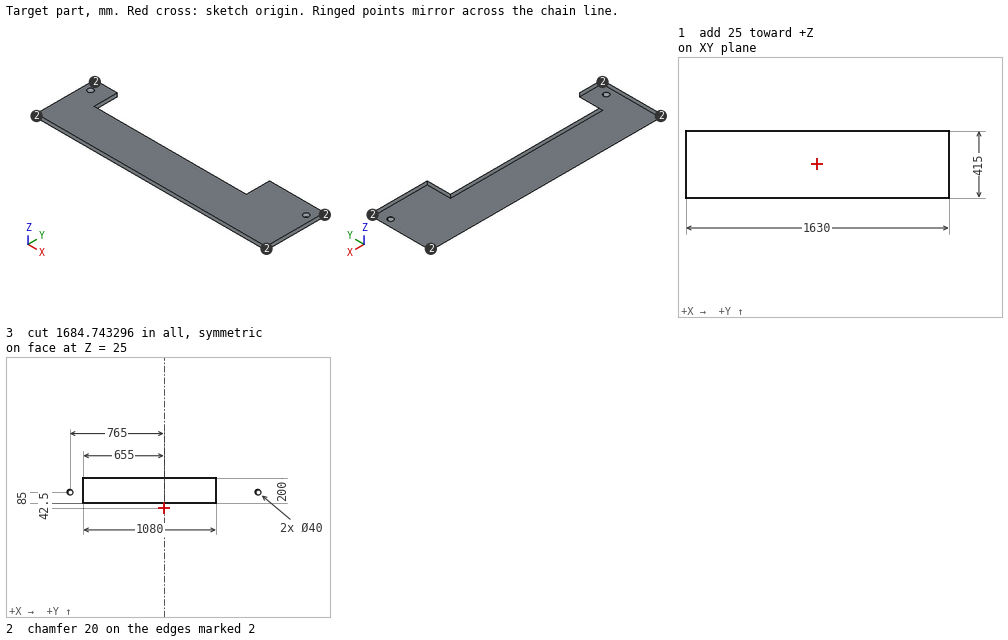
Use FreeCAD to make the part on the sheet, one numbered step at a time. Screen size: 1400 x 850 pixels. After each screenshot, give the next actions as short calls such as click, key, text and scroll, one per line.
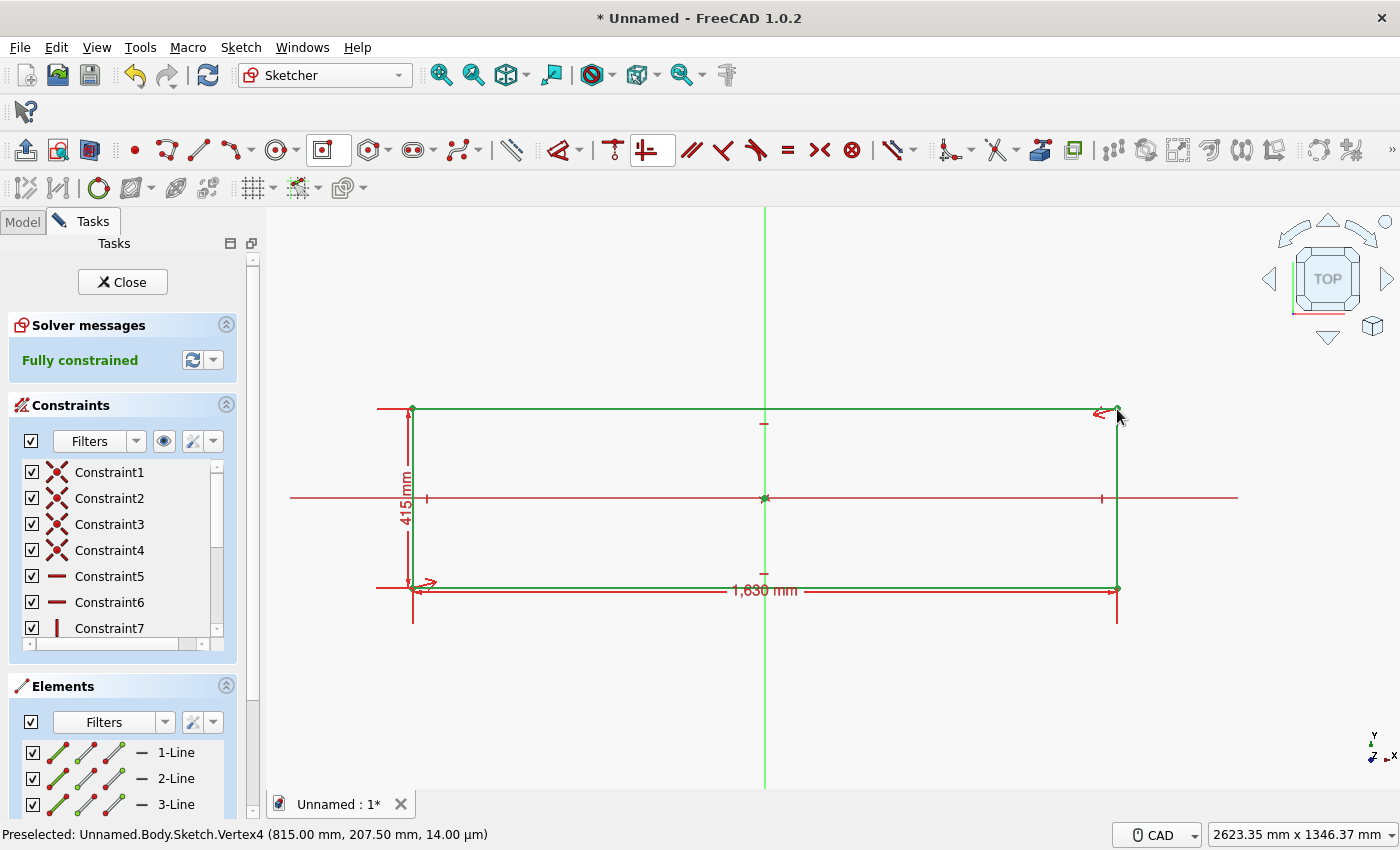
click(123, 282)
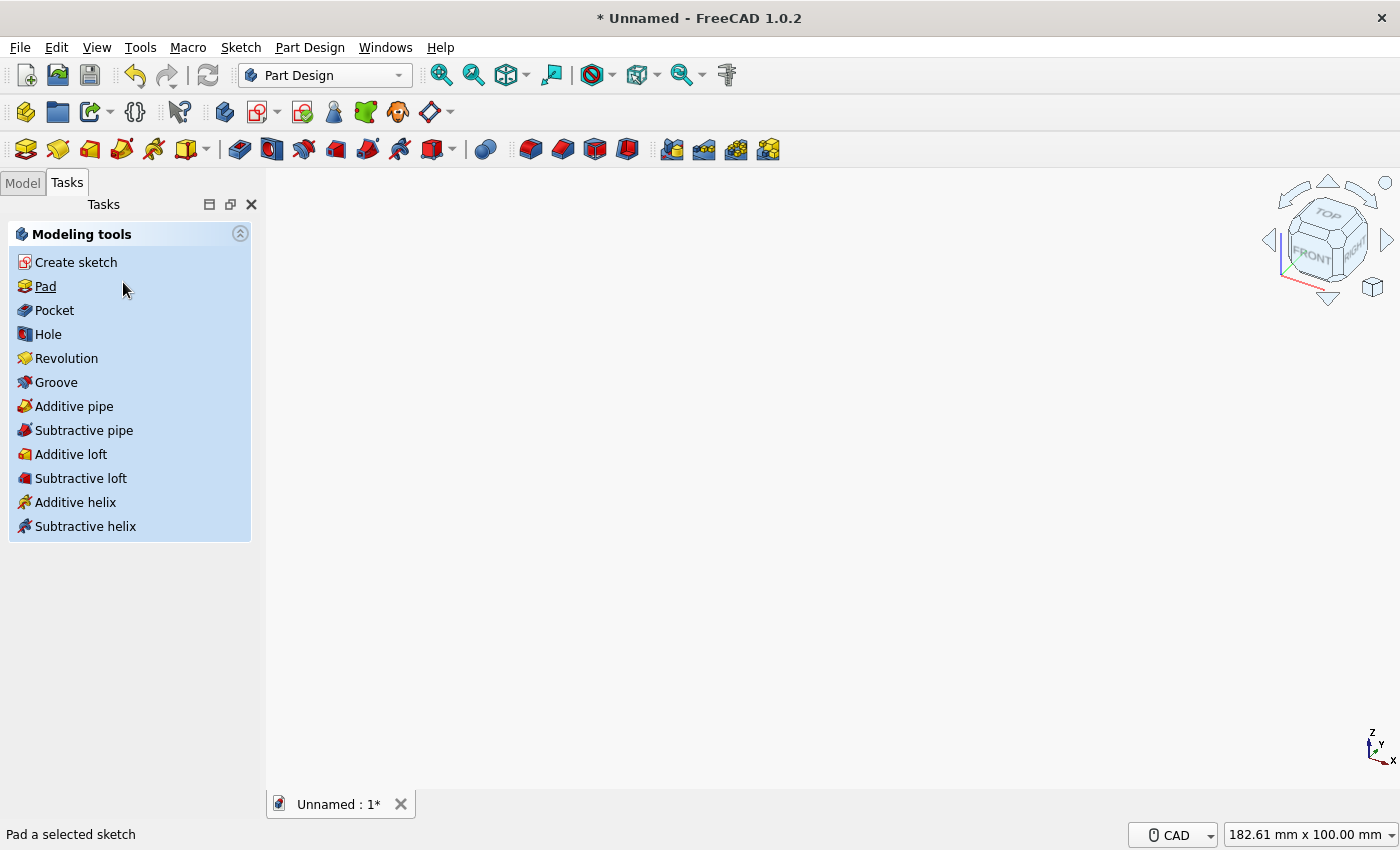
click(26, 150)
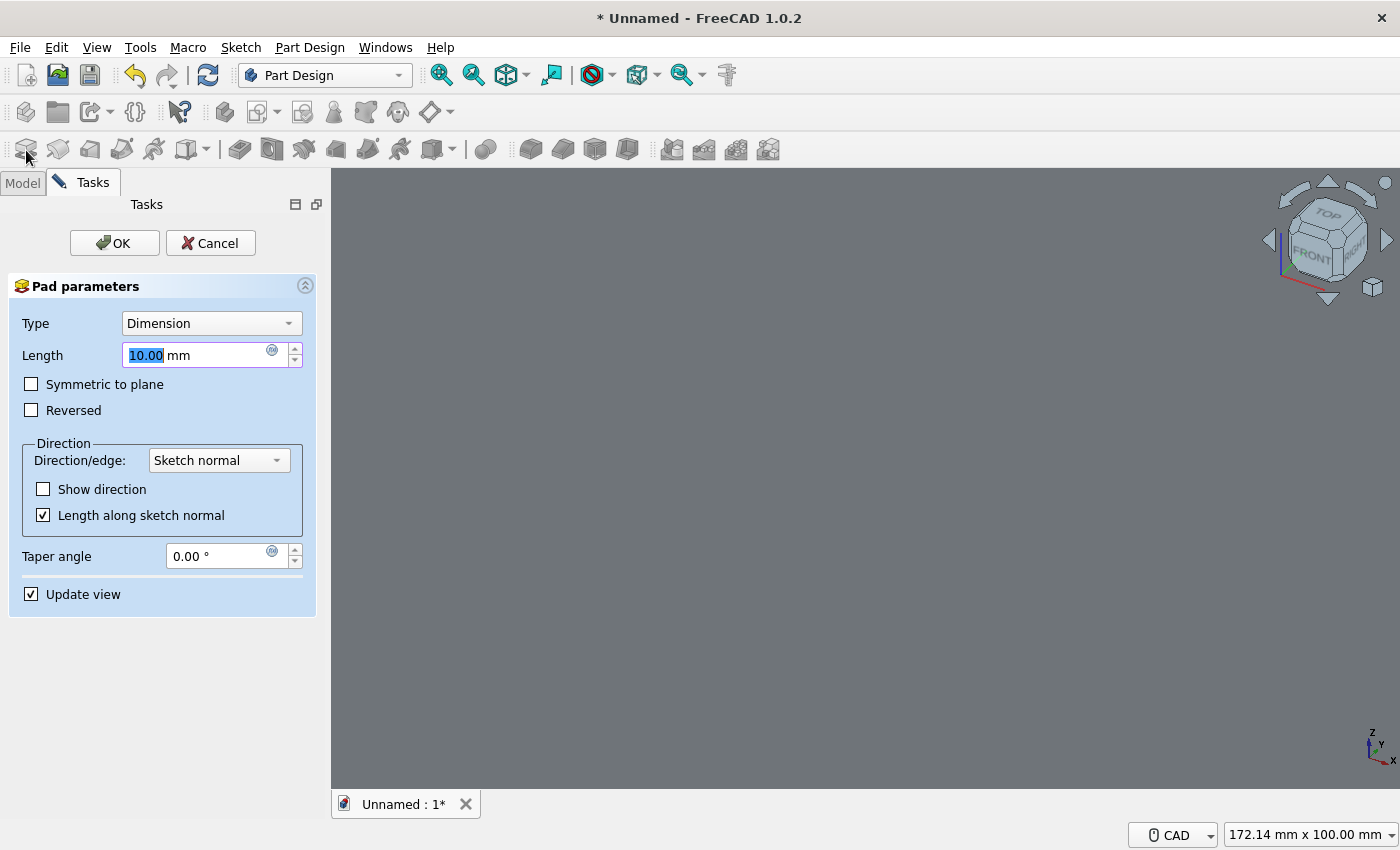
text(25)
key(Tab)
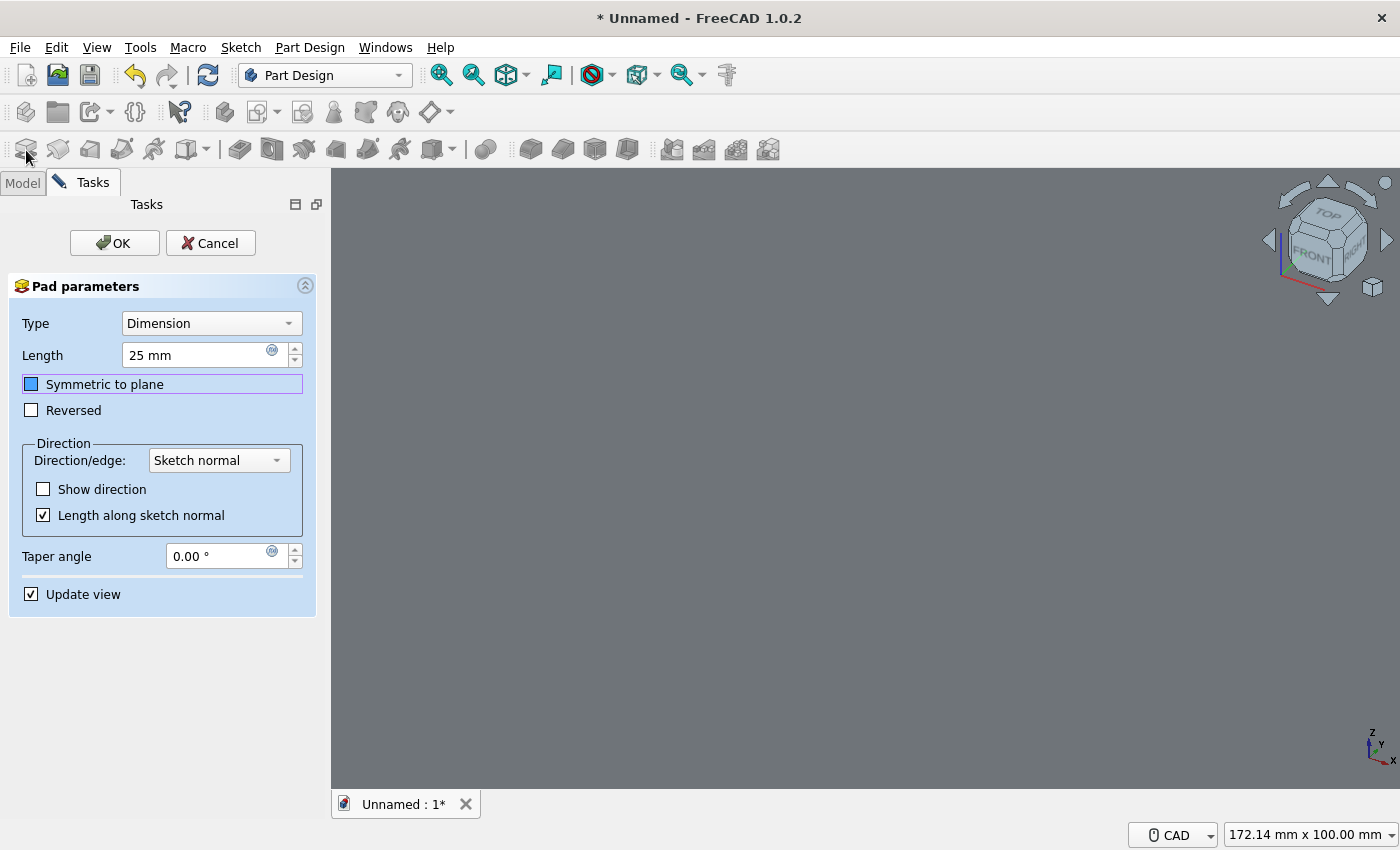
click(115, 243)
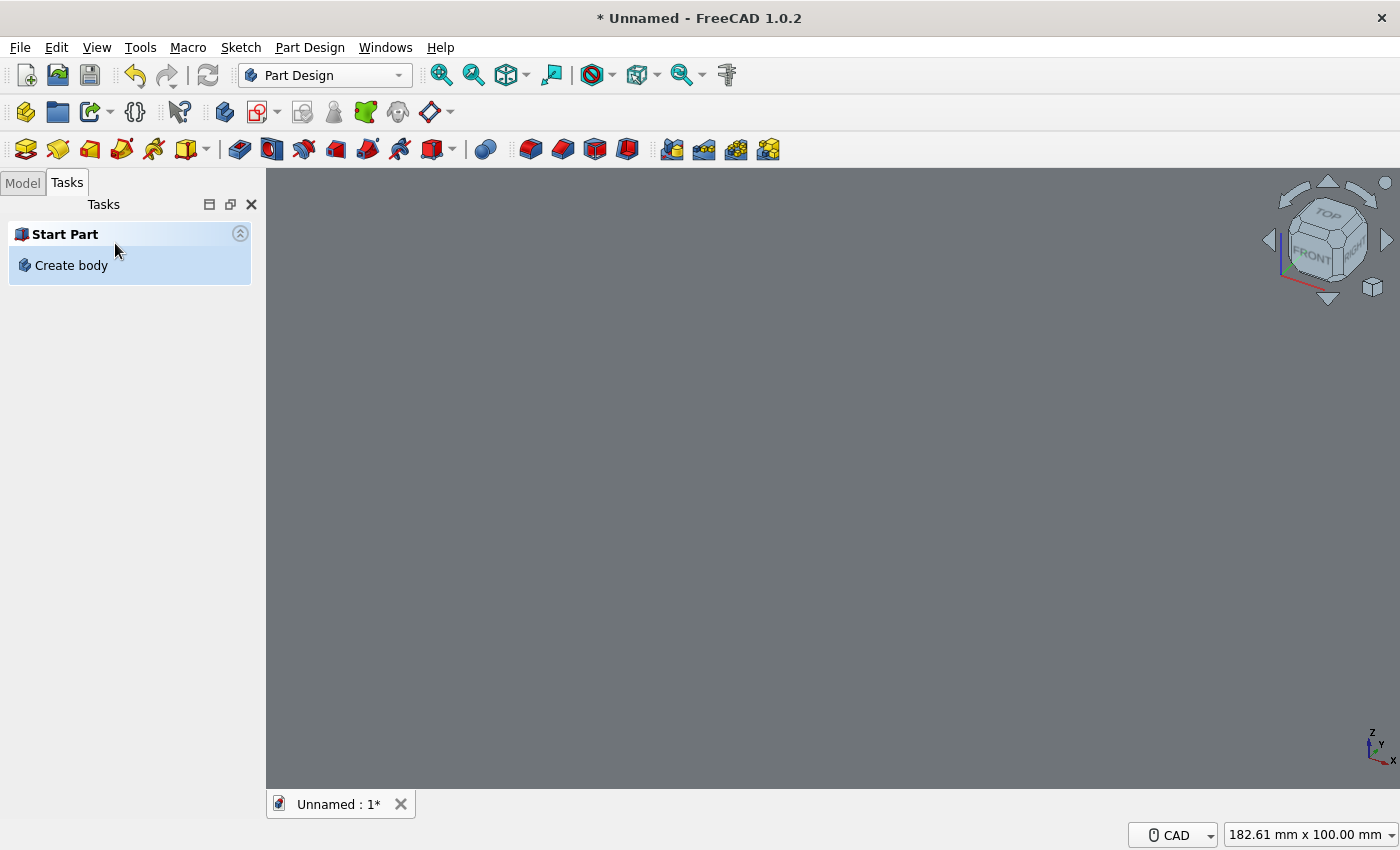
click(442, 76)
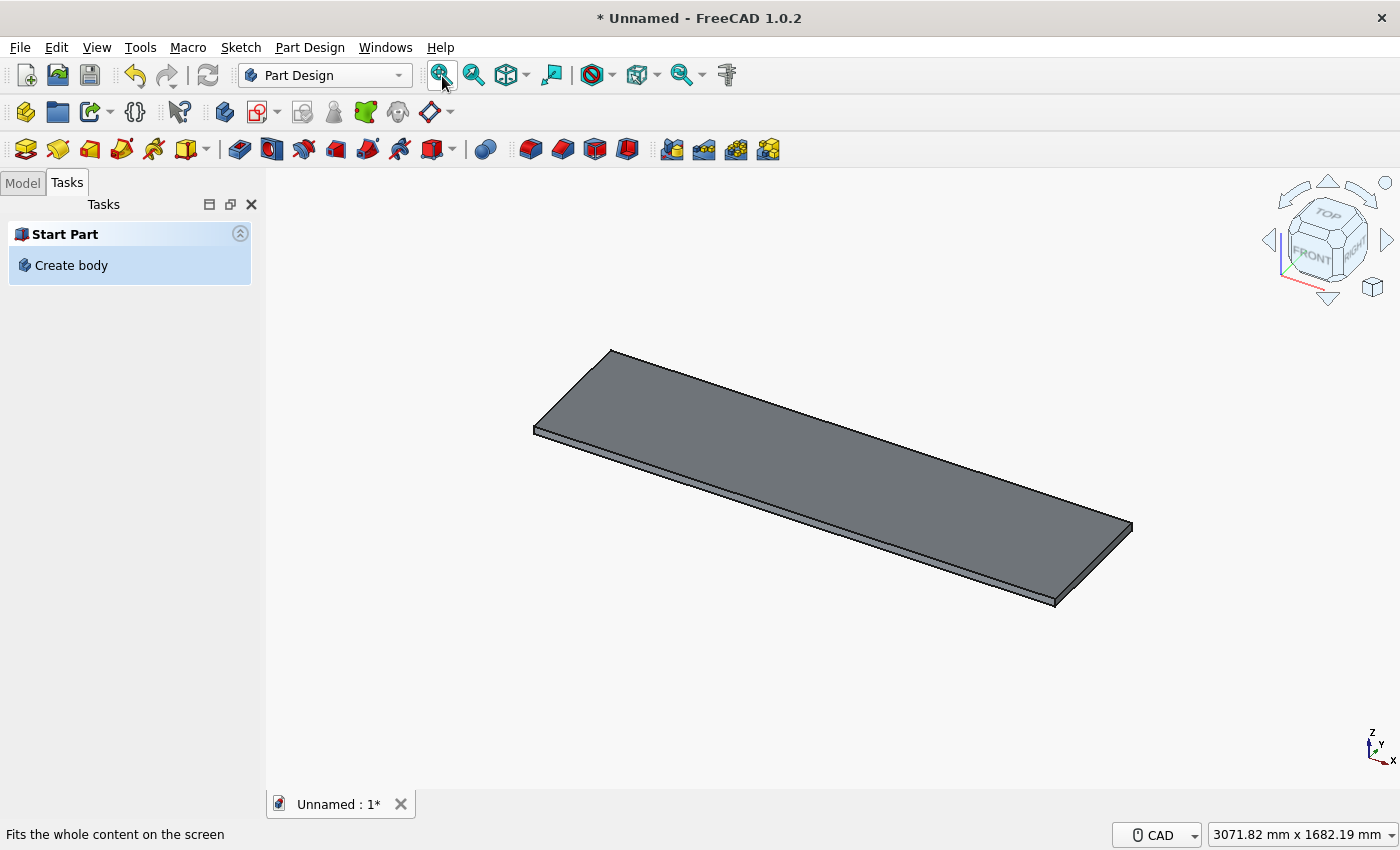
scroll(611, 353, up, 8)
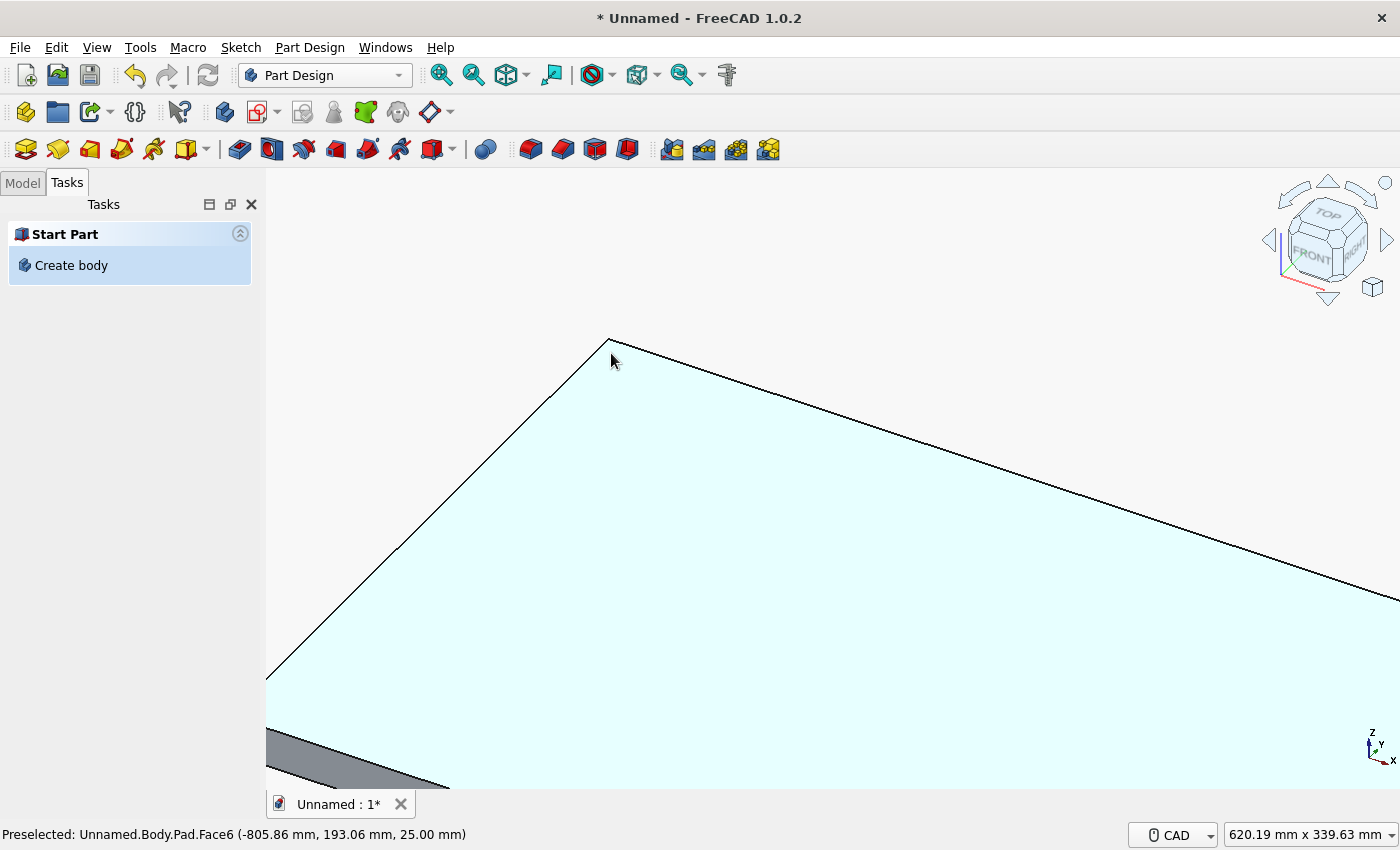
click(442, 76)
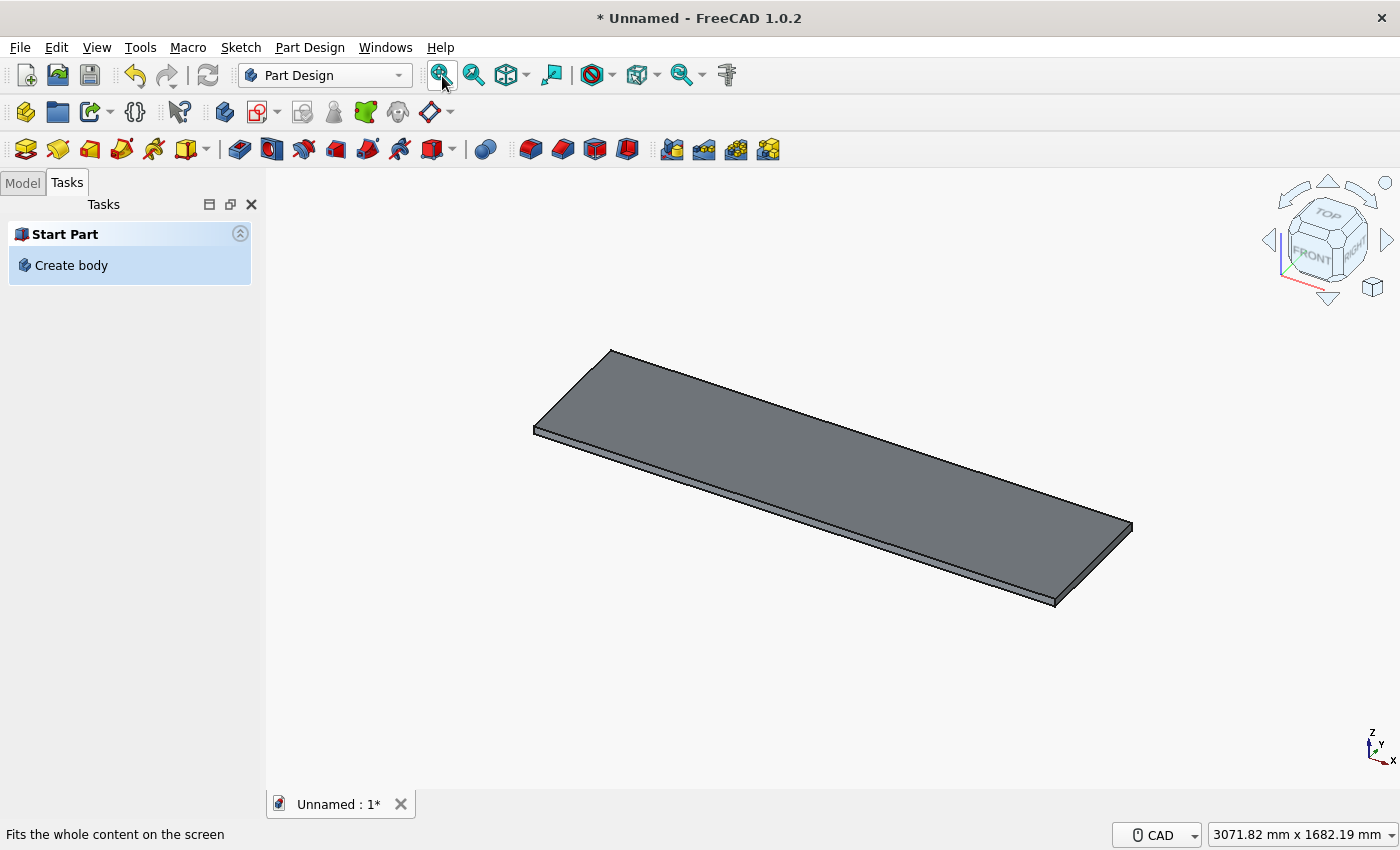
key(0)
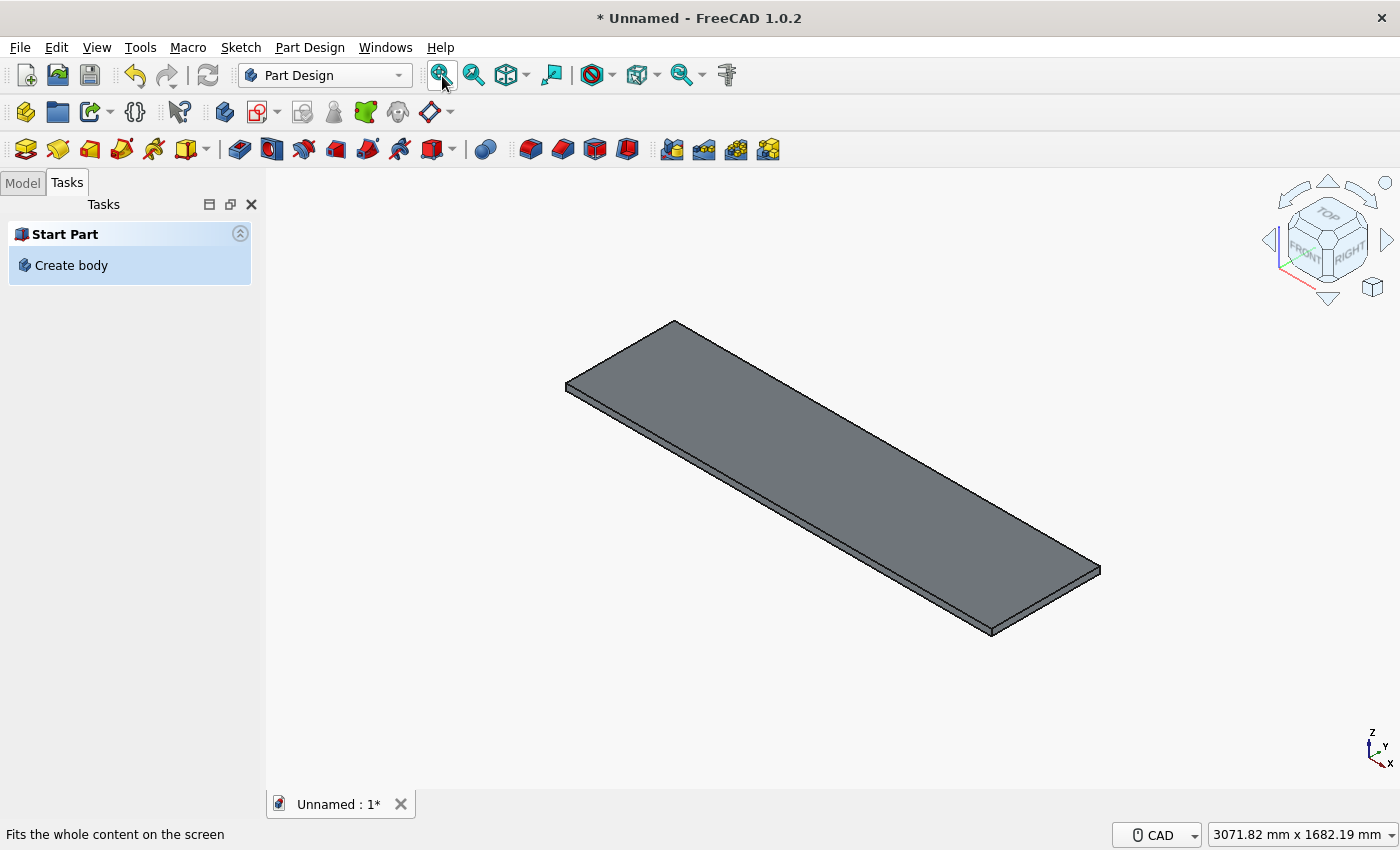
click(992, 634)